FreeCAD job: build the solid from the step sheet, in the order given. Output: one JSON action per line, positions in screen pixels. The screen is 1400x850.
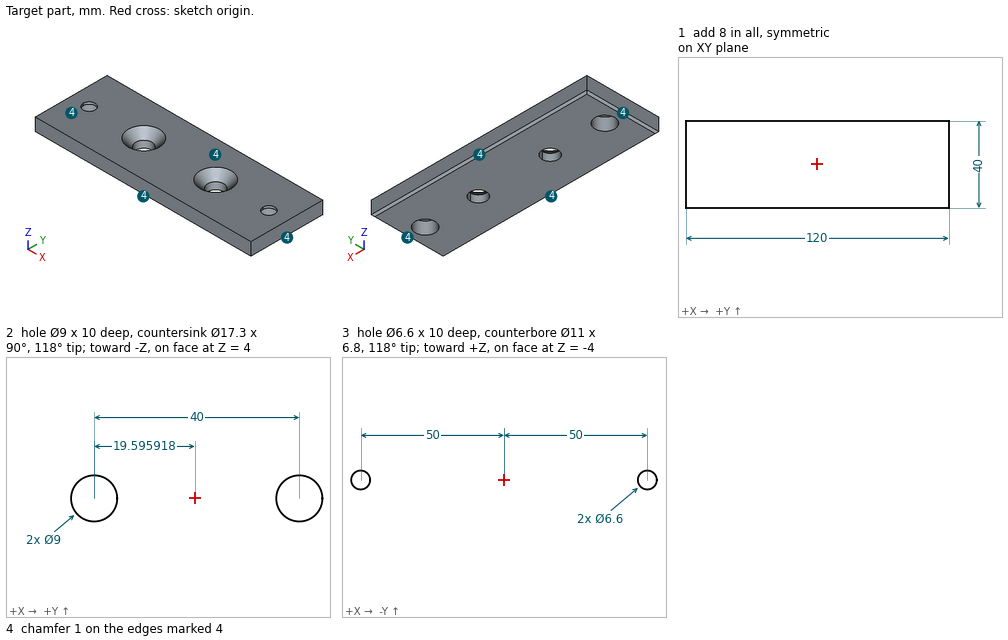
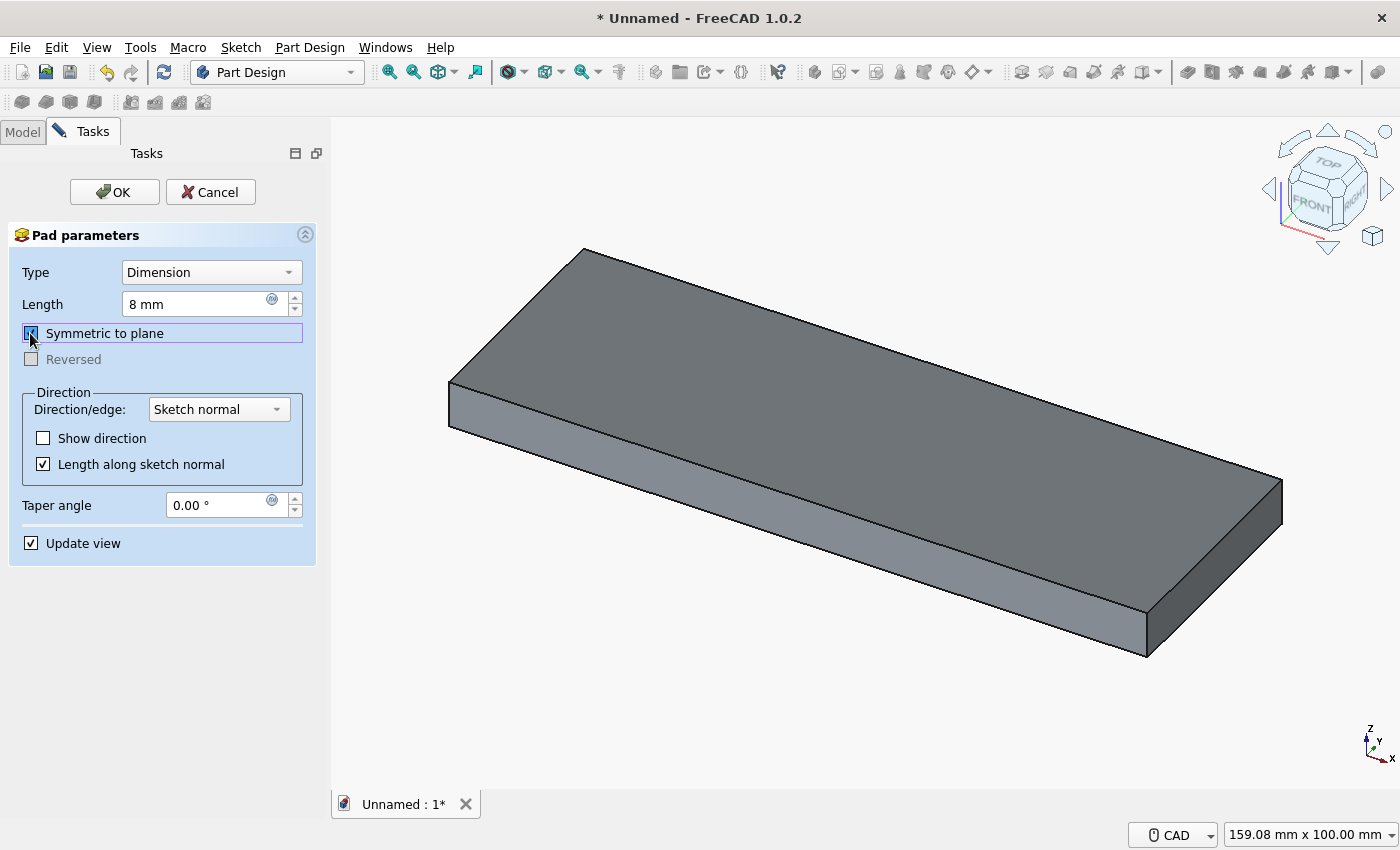
{"action": "left_click", "coordinate": [115, 192]}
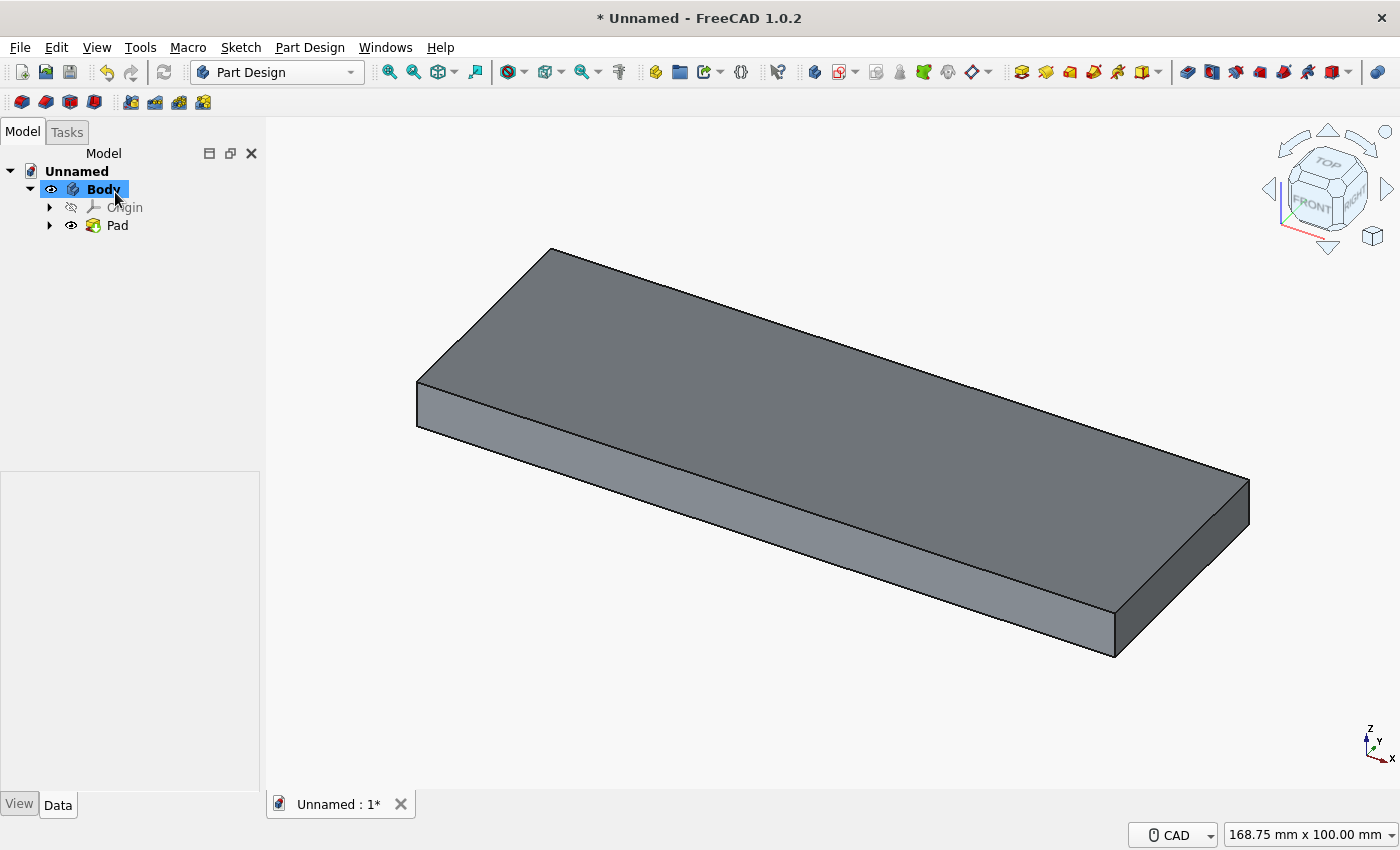
{"action": "left_click", "coordinate": [1033, 496]}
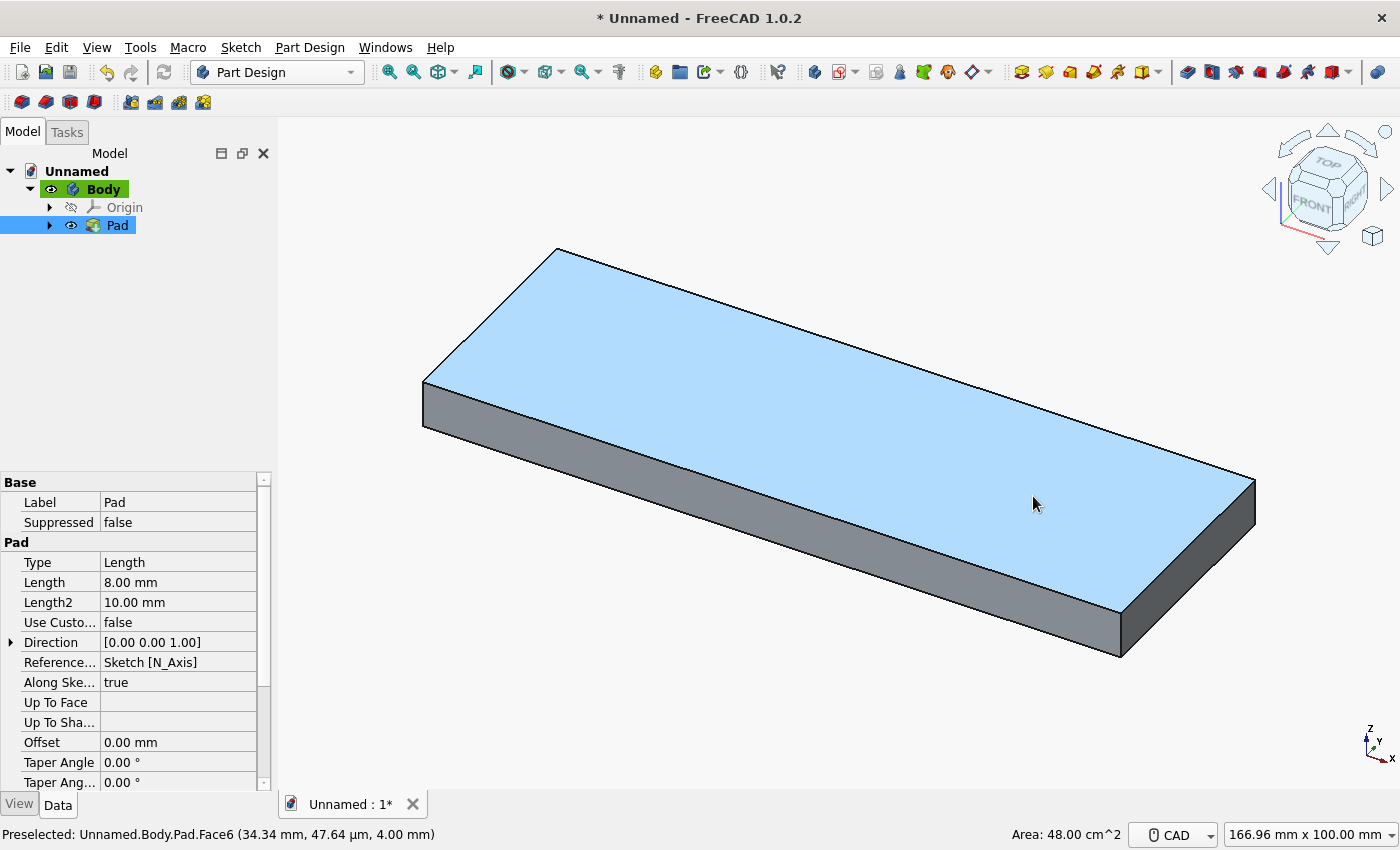
{"action": "left_click", "coordinate": [840, 72]}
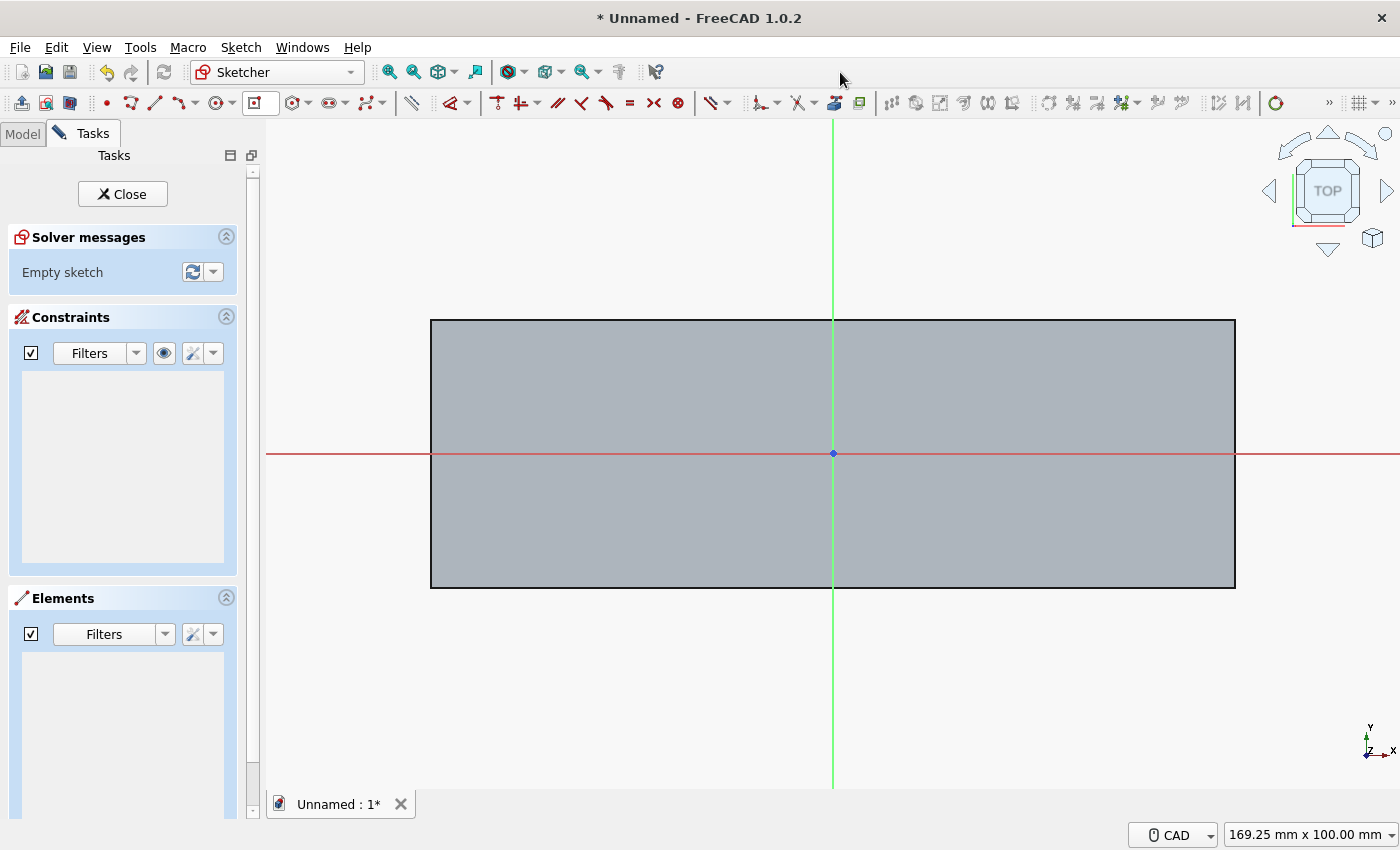
{"action": "scroll", "coordinate": [894, 454], "scroll_direction": "up", "scroll_amount": 4}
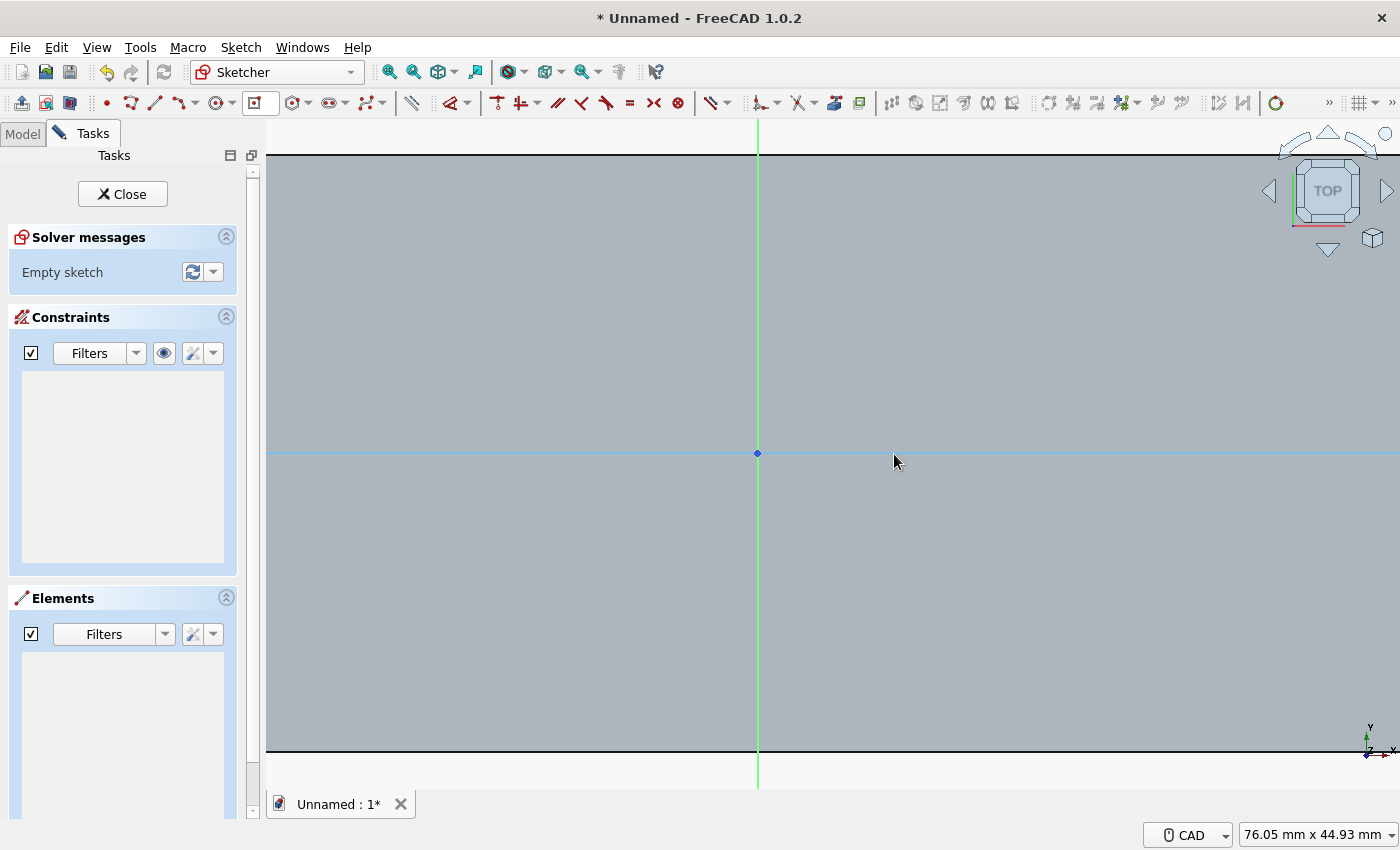
{"action": "key", "text": "g c"}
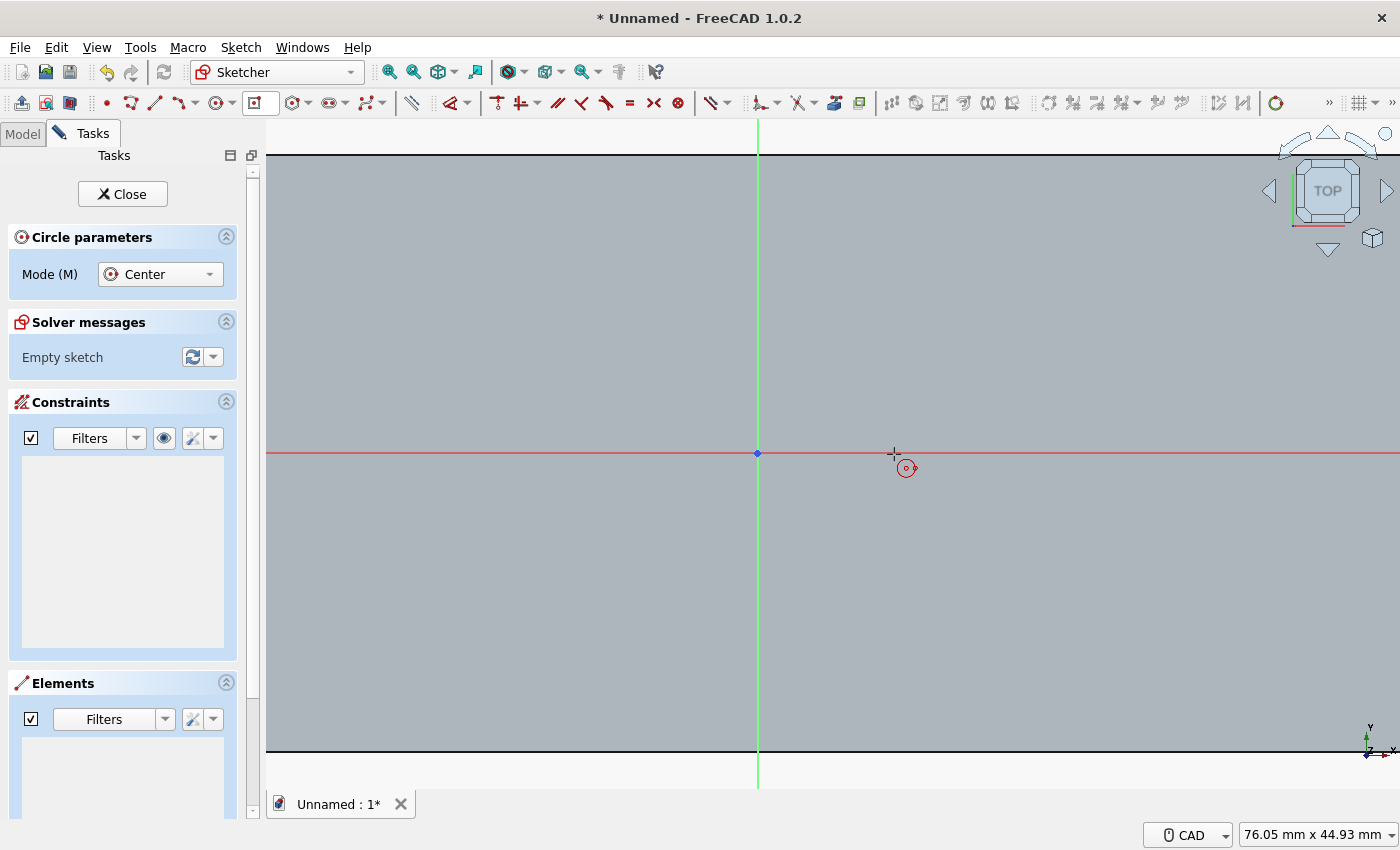
{"action": "left_click", "coordinate": [465, 453]}
{"action": "left_click", "coordinate": [513, 406]}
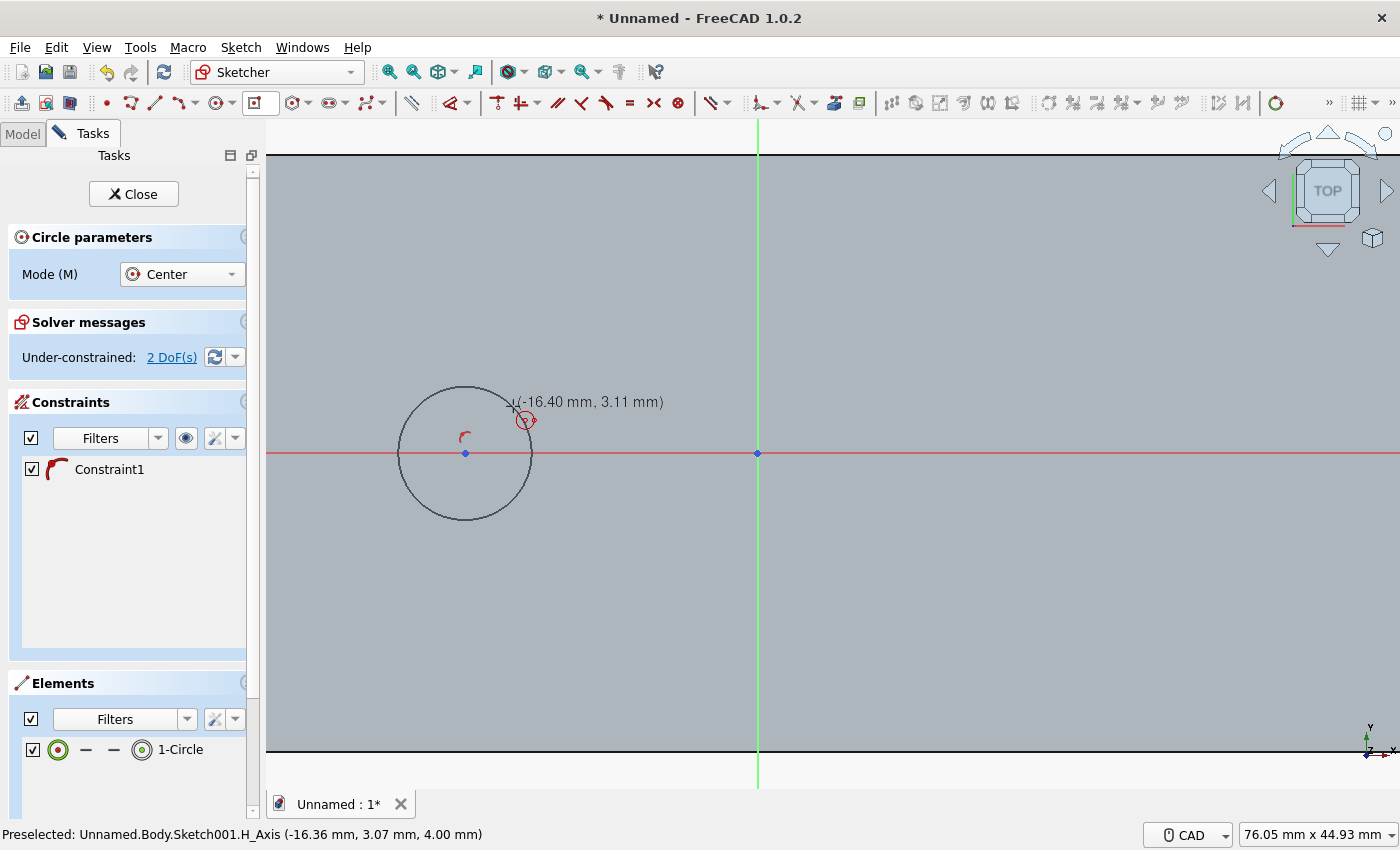
{"action": "left_click", "coordinate": [1062, 453]}
{"action": "left_click", "coordinate": [1109, 406]}
{"action": "key", "text": "Escape"}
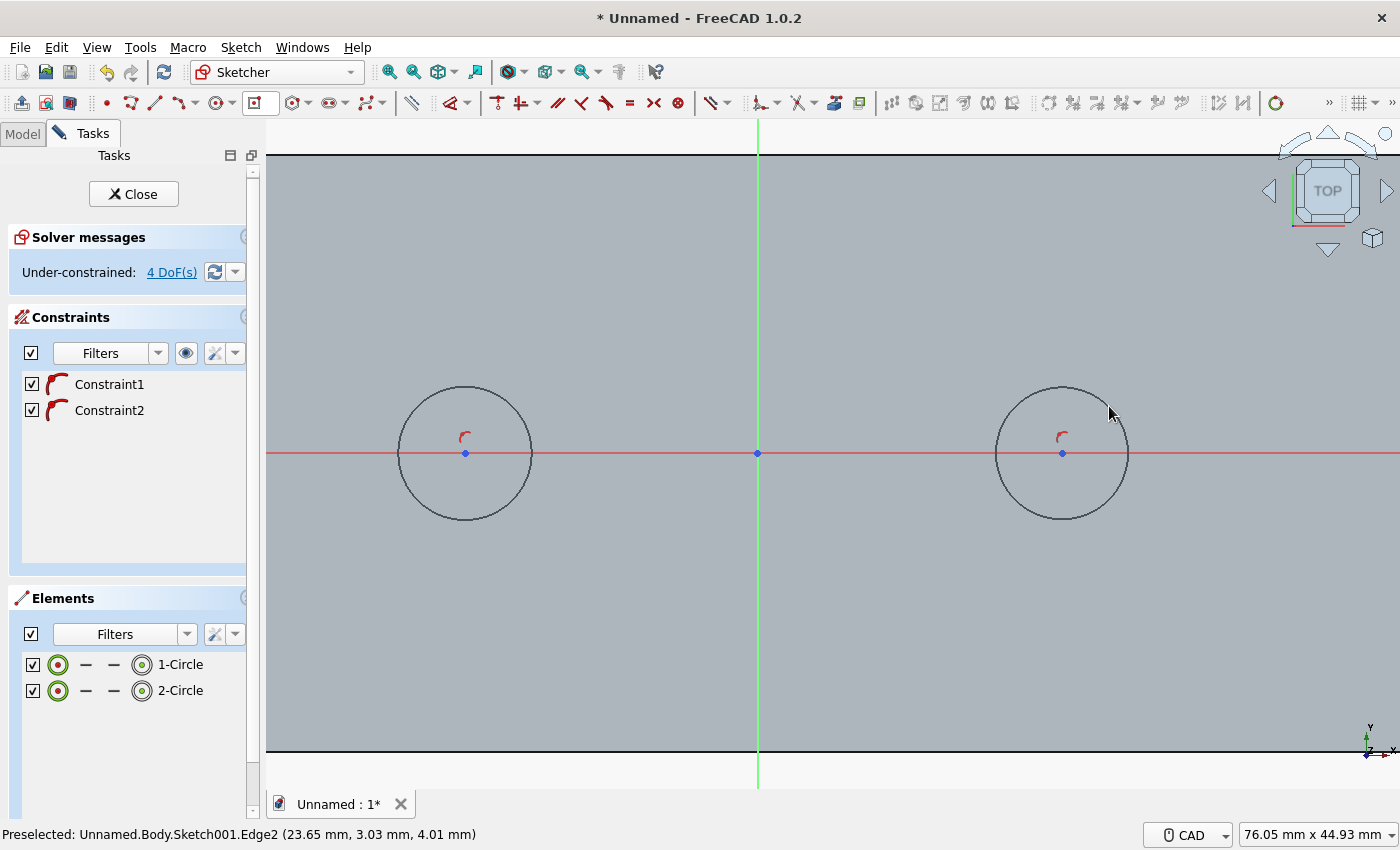
{"action": "left_click", "coordinate": [512, 406]}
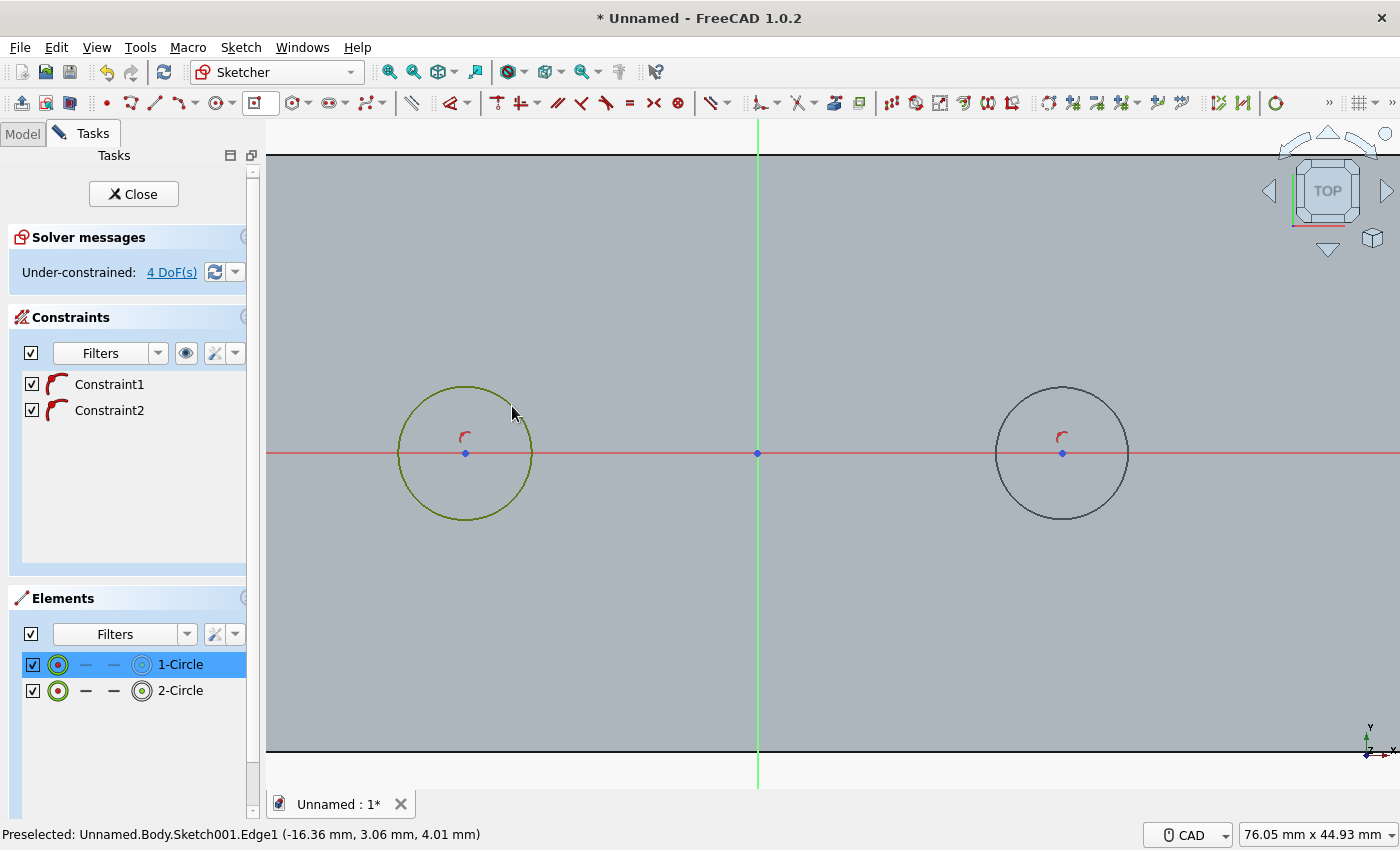
{"action": "left_click", "coordinate": [1109, 407]}